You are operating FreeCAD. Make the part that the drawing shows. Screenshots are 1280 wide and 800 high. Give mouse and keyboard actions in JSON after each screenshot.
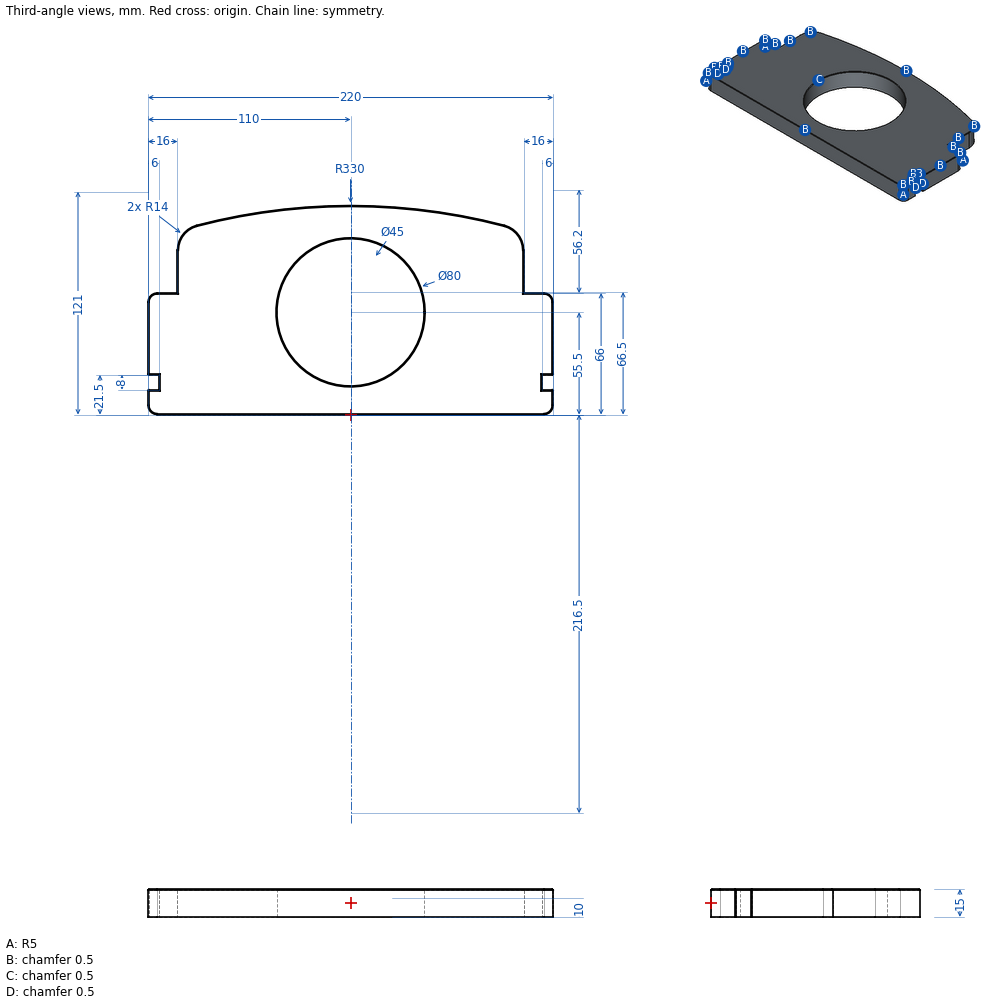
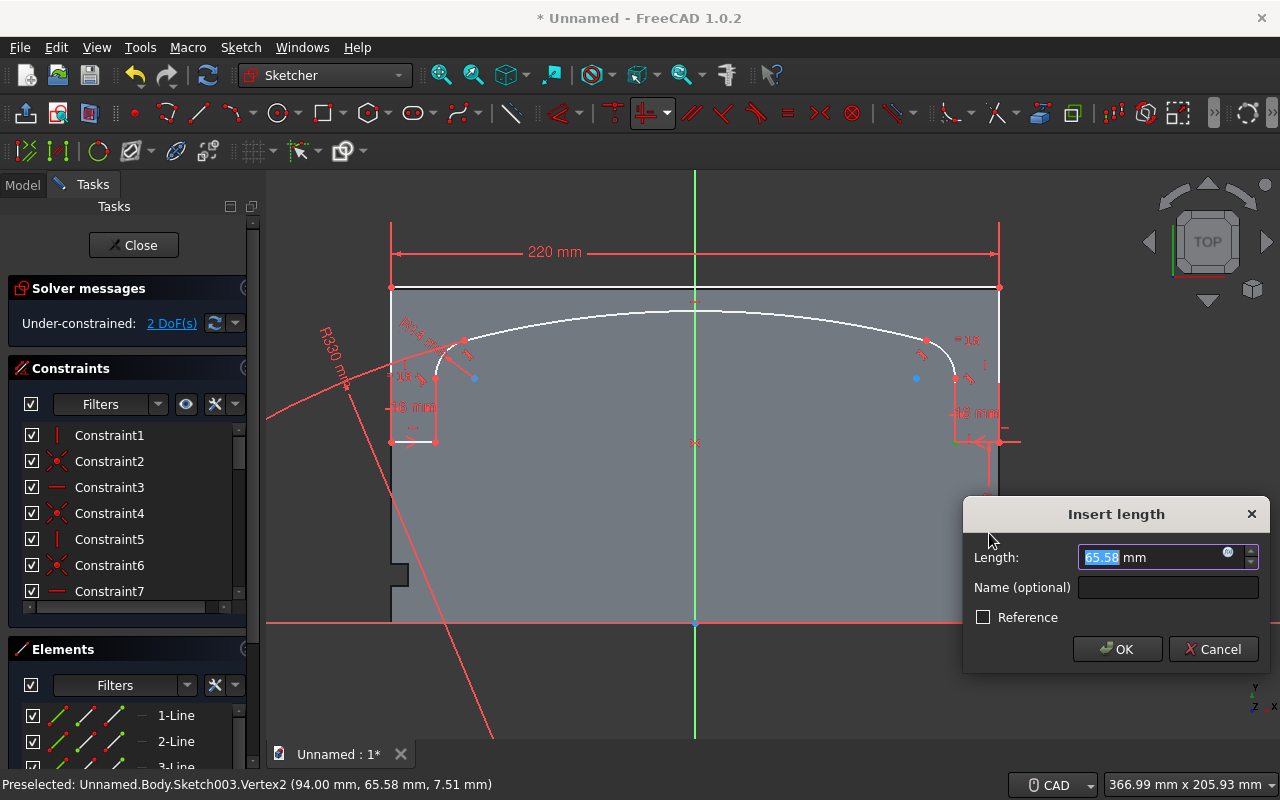
{"action": "type", "text": "66"}
{"action": "key", "text": "Return"}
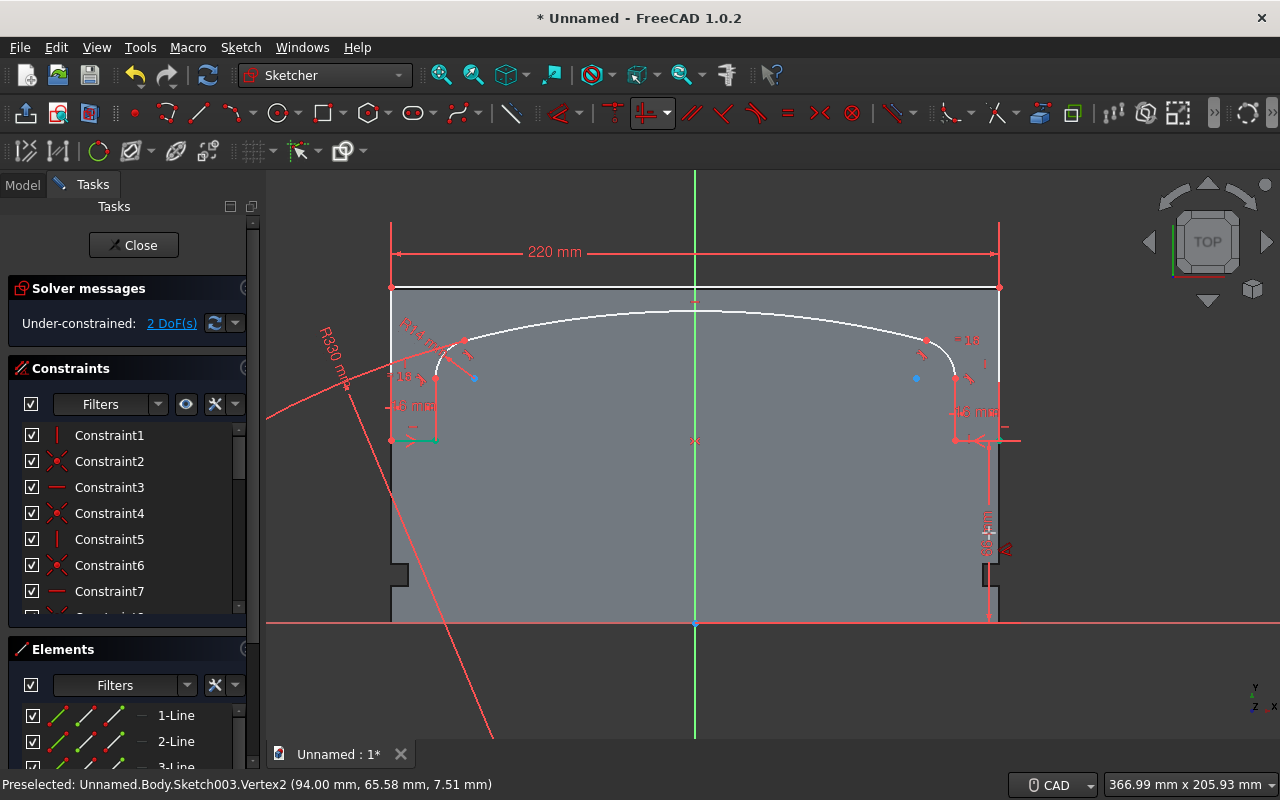
{"action": "left_click", "coordinate": [999, 395]}
{"action": "left_click", "coordinate": [1033, 364]}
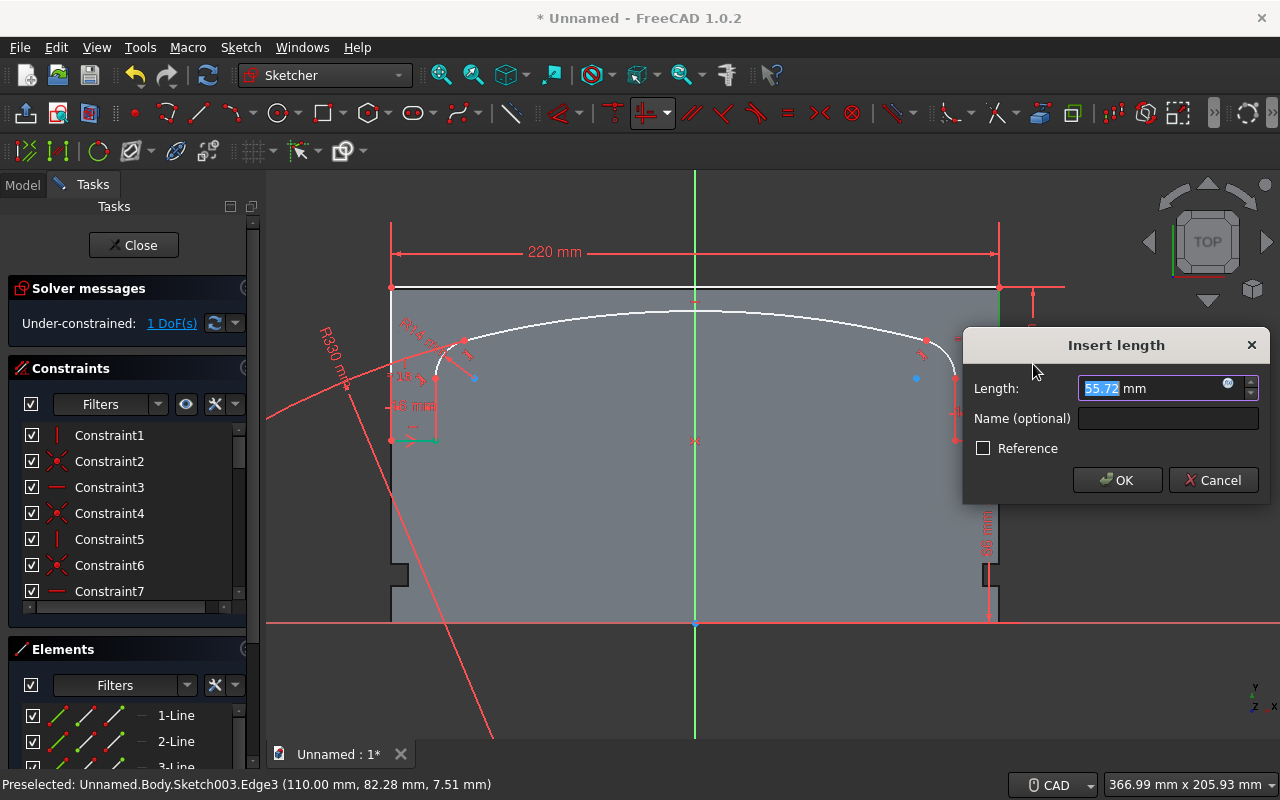
{"action": "type", "text": "56.2"}
{"action": "key", "text": "Return"}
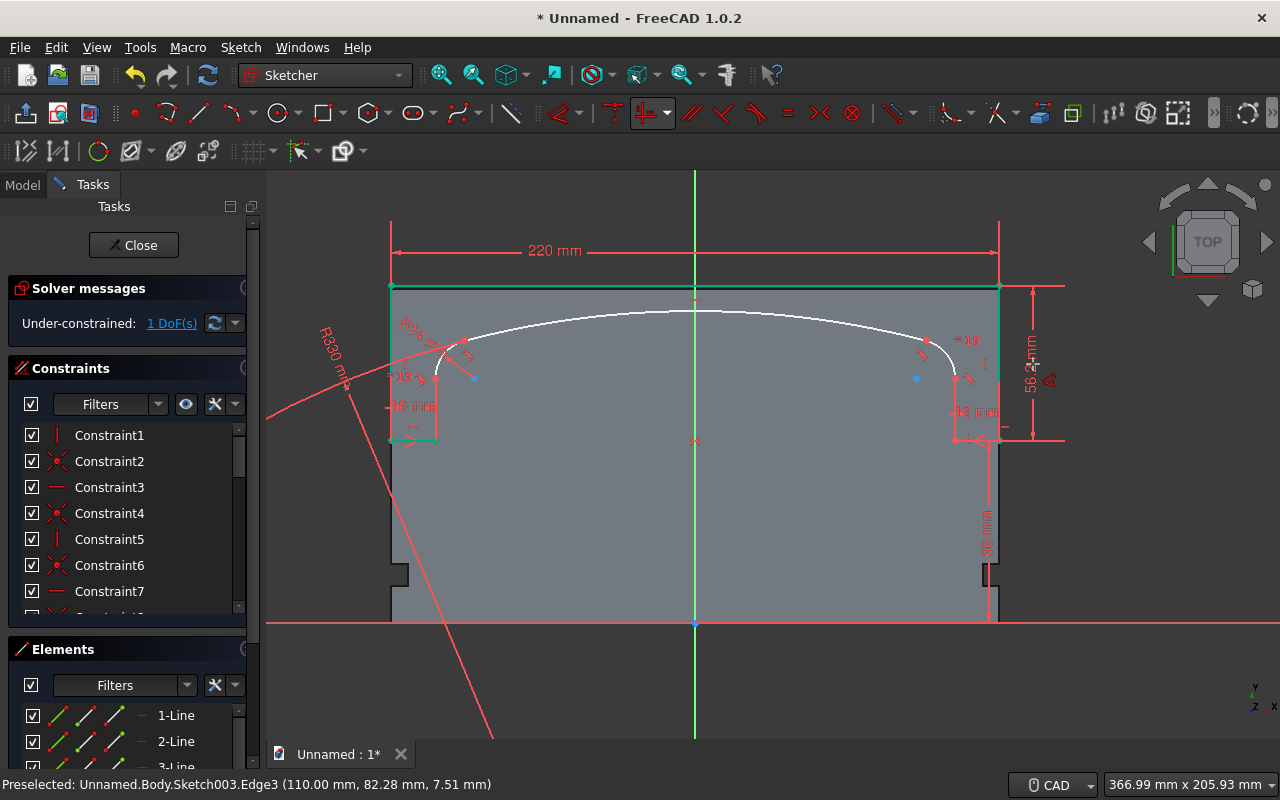
{"action": "scroll", "coordinate": [710, 280], "scroll_direction": "down", "scroll_amount": 5}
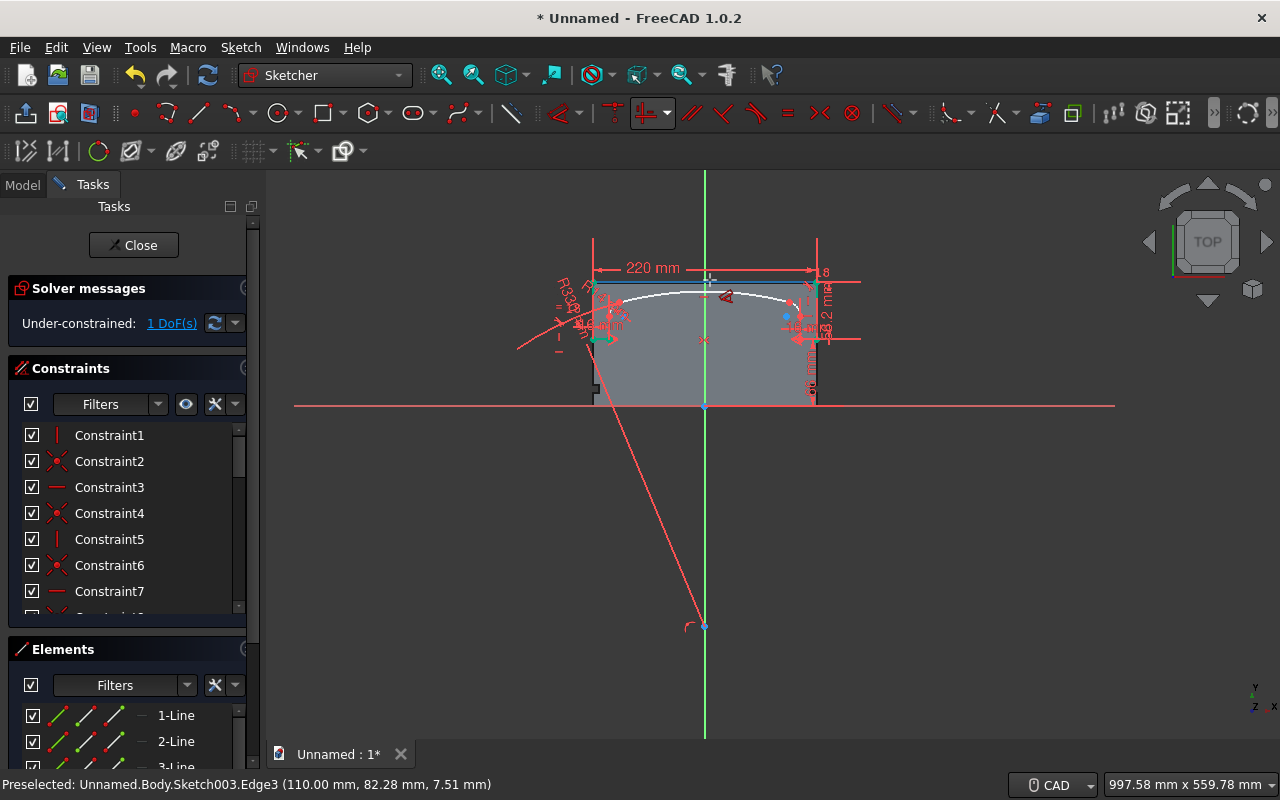
{"action": "left_click", "coordinate": [705, 627]}
{"action": "left_click", "coordinate": [739, 517]}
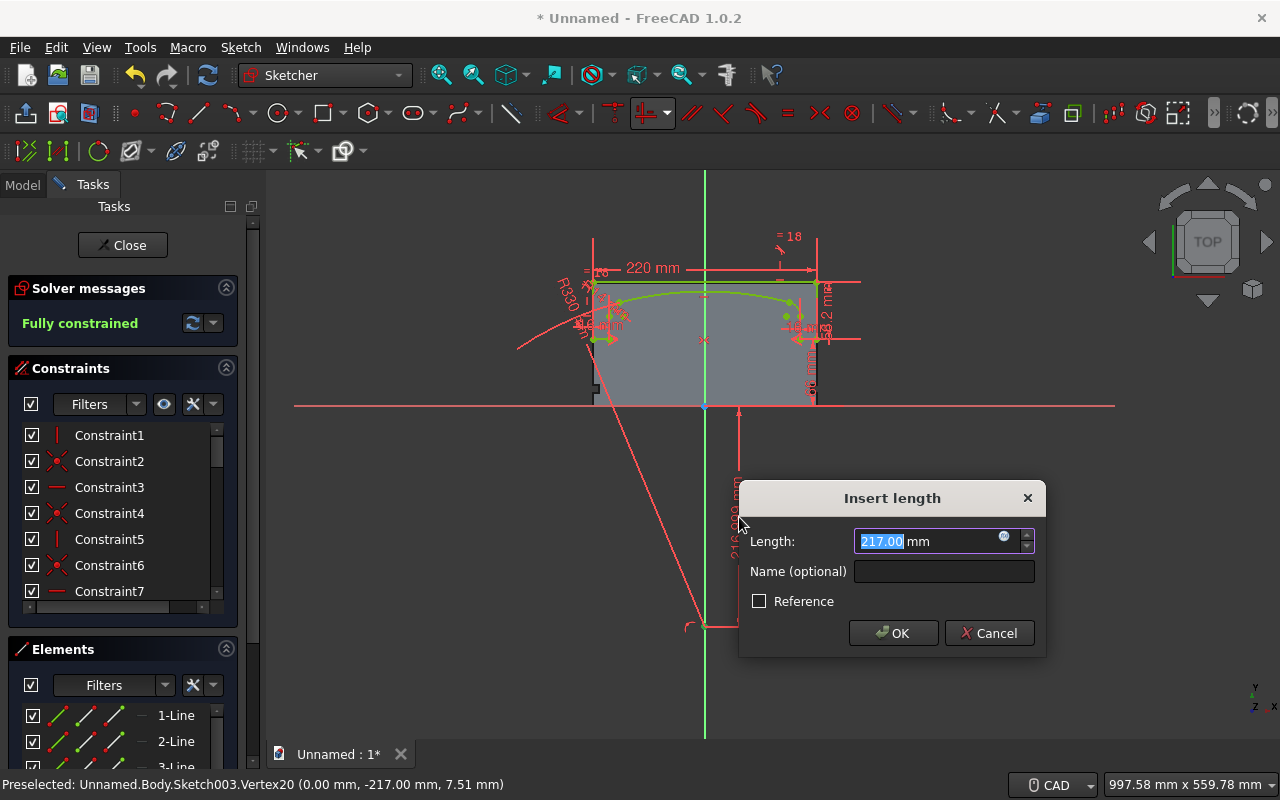
{"action": "type", "text": "216.5"}
{"action": "key", "text": "Return"}
{"action": "key", "text": "Escape"}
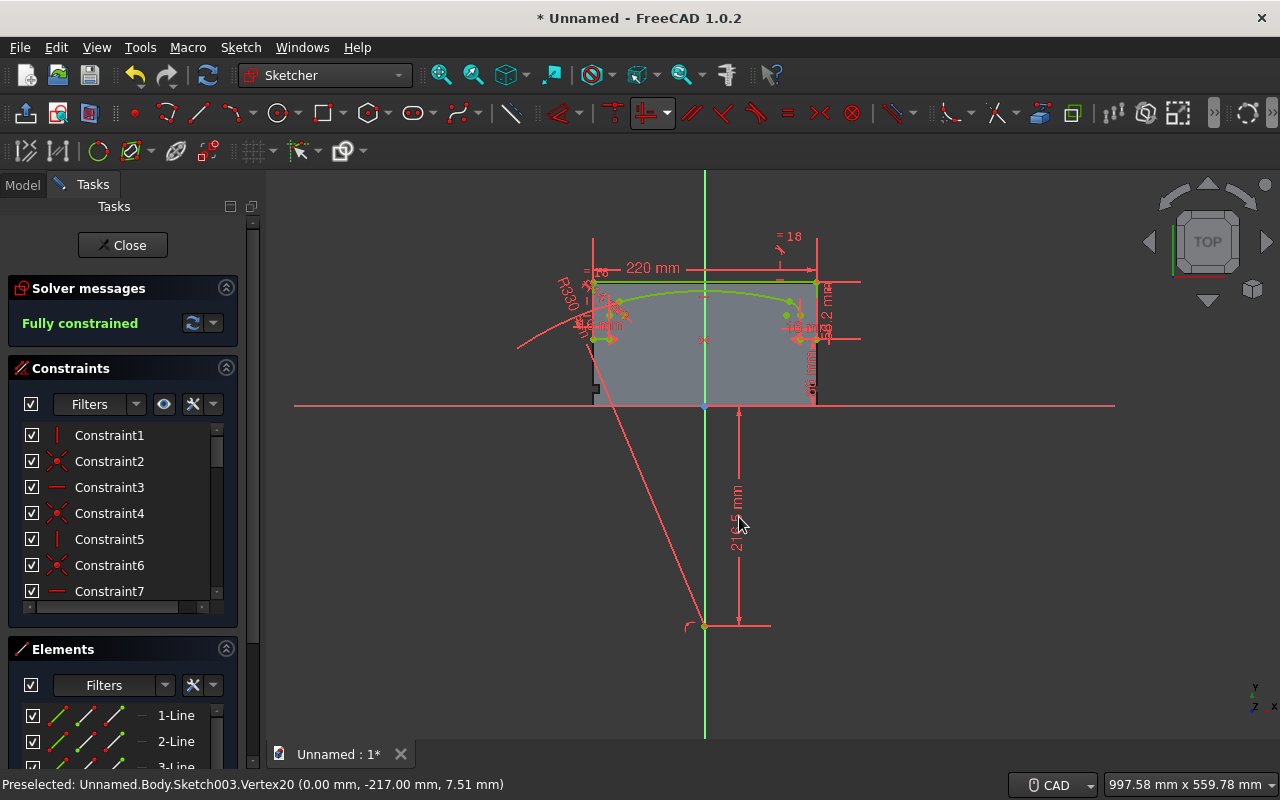
{"action": "left_click", "coordinate": [123, 245]}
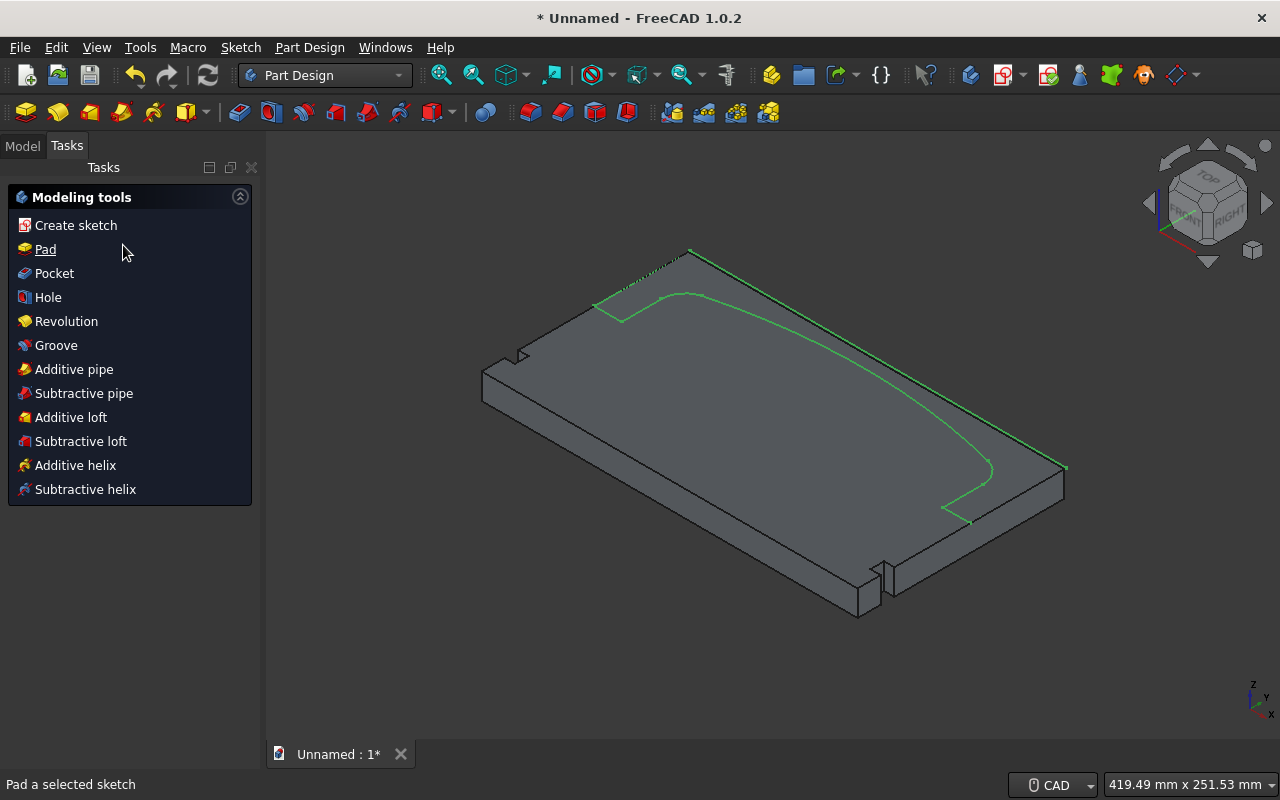
{"action": "left_click", "coordinate": [240, 112]}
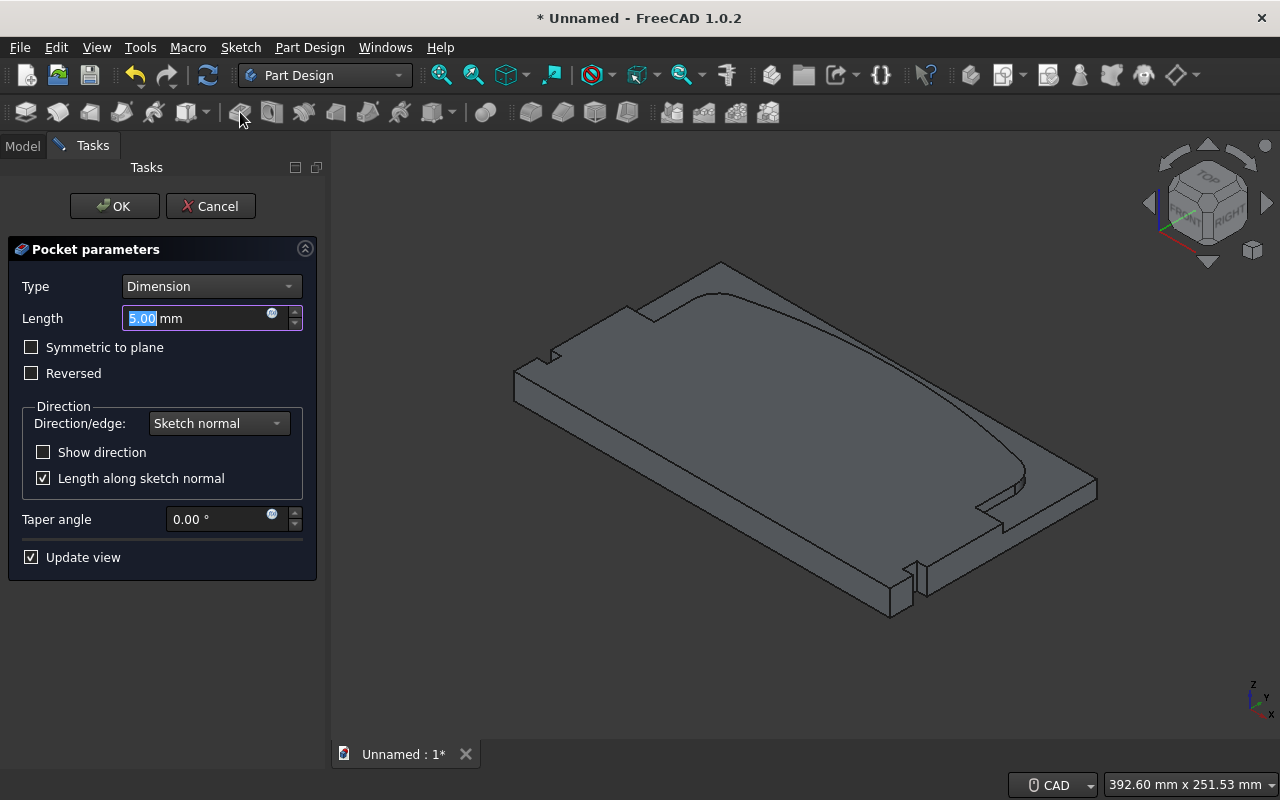
{"action": "left_click", "coordinate": [212, 286]}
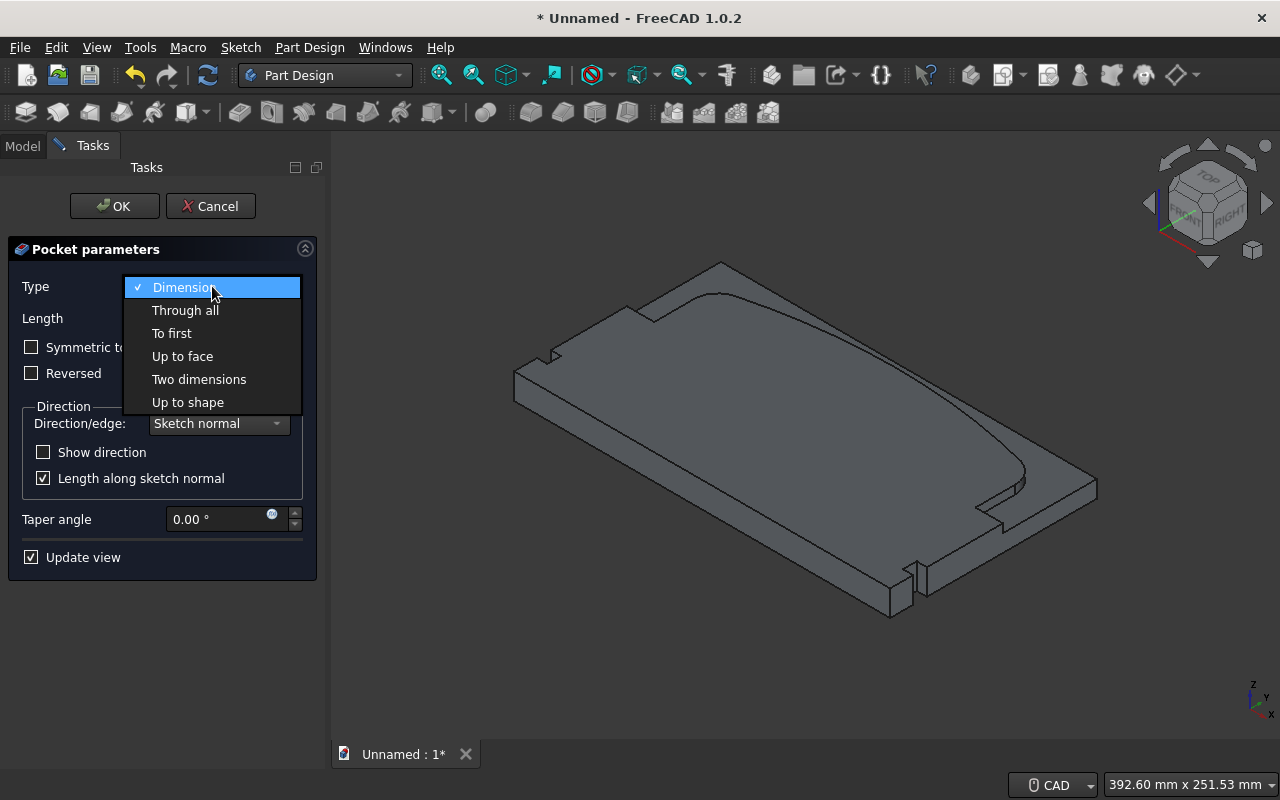
{"action": "left_click", "coordinate": [212, 310]}